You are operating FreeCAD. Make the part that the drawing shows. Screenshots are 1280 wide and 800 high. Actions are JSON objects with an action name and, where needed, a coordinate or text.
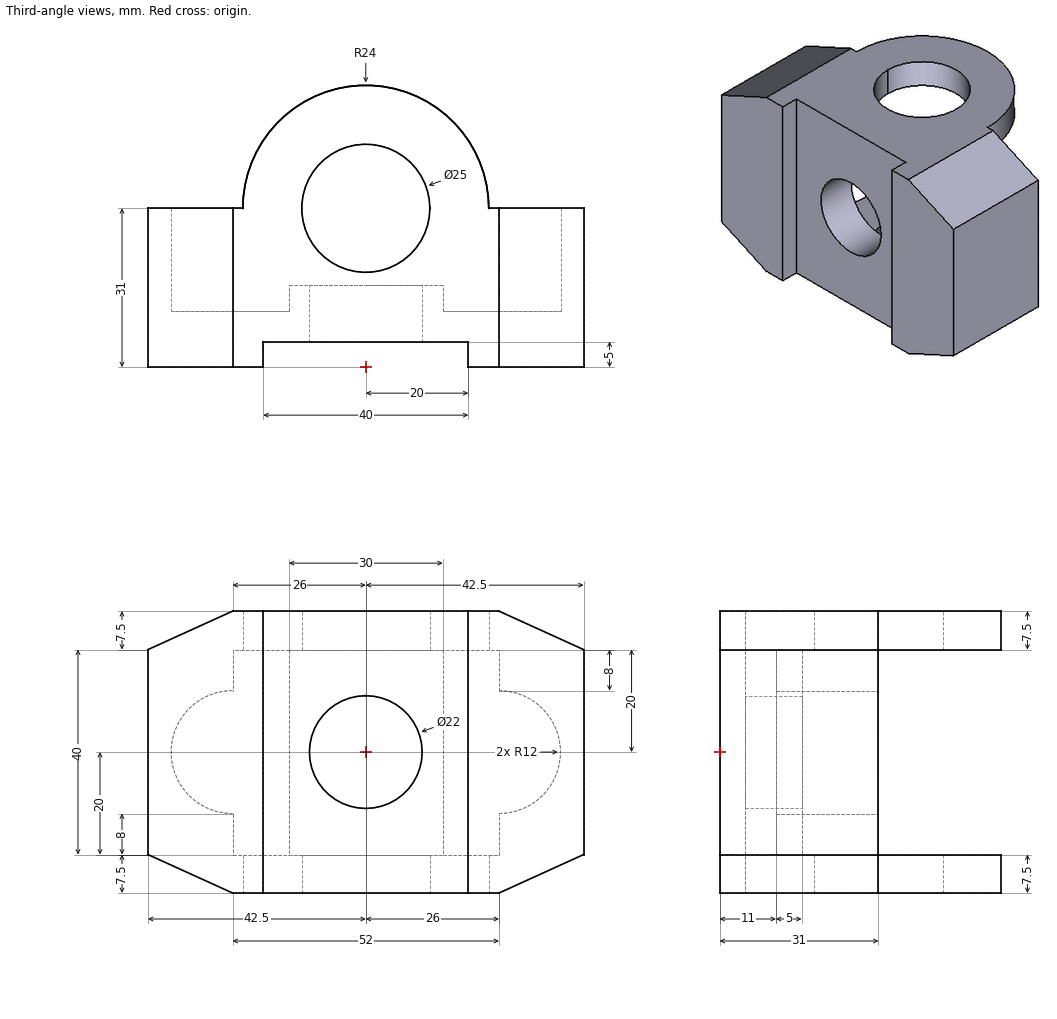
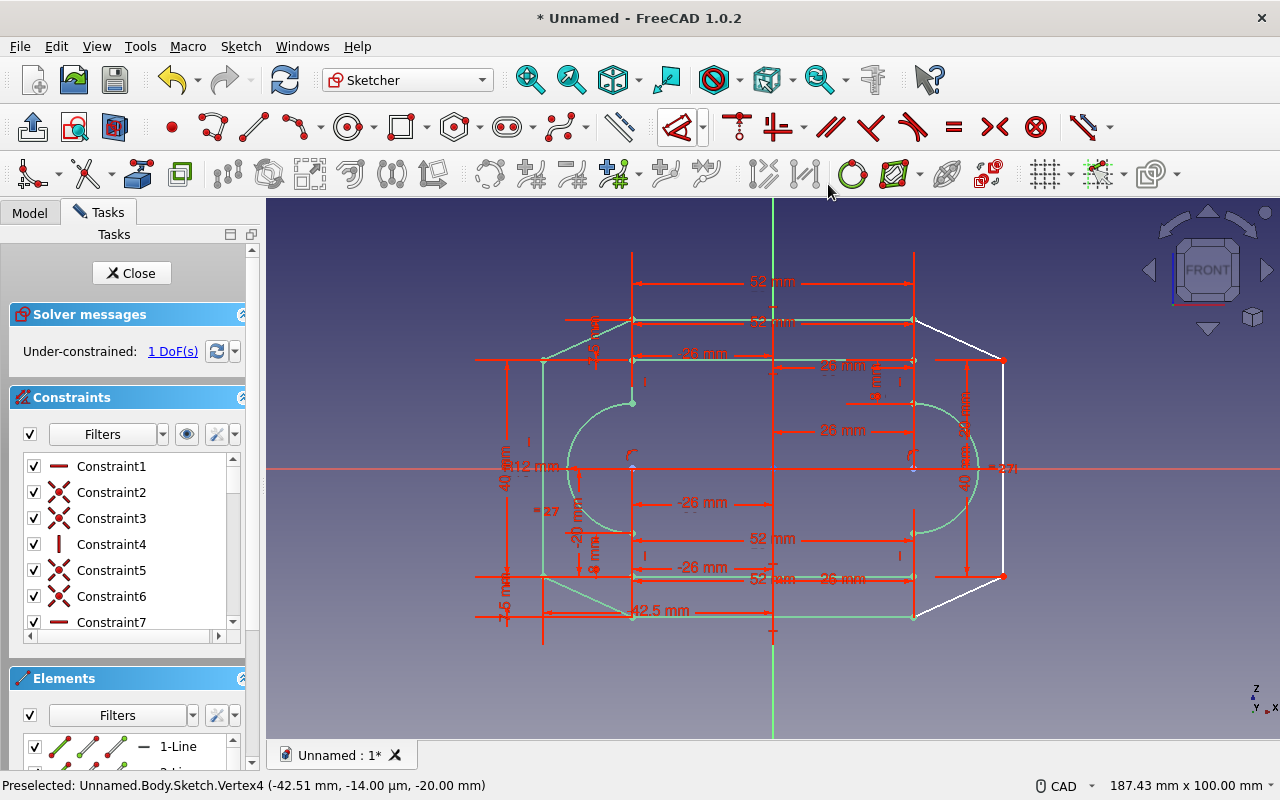
{"action": "left_click", "coordinate": [1003, 360]}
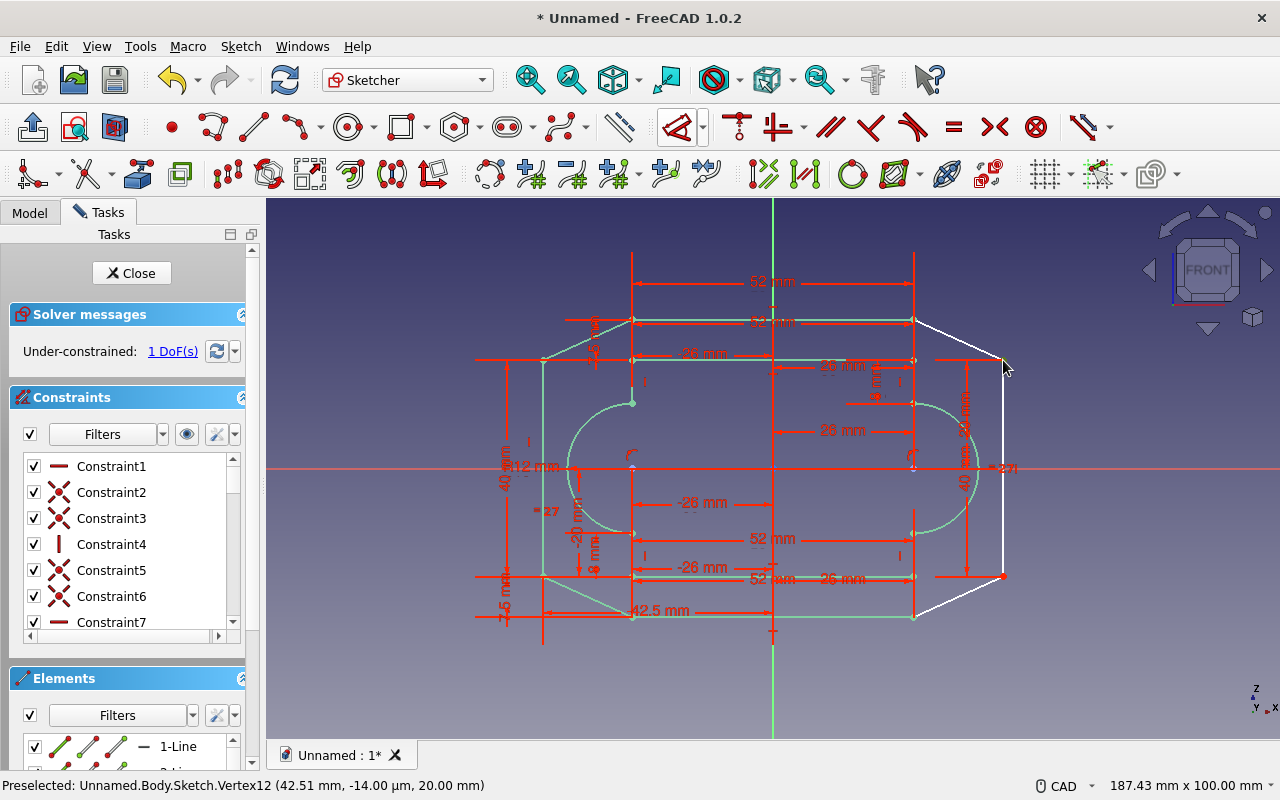
{"action": "left_click", "coordinate": [702, 128]}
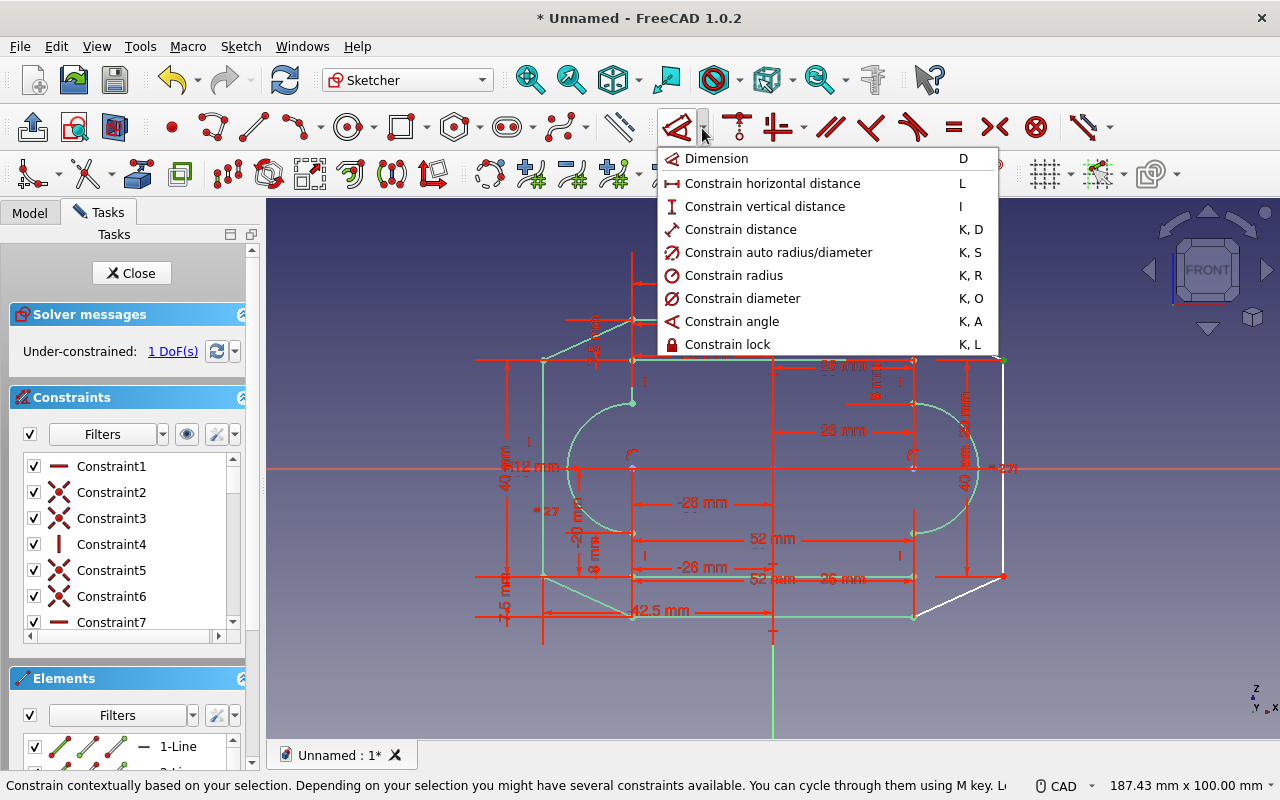
{"action": "left_click", "coordinate": [828, 184]}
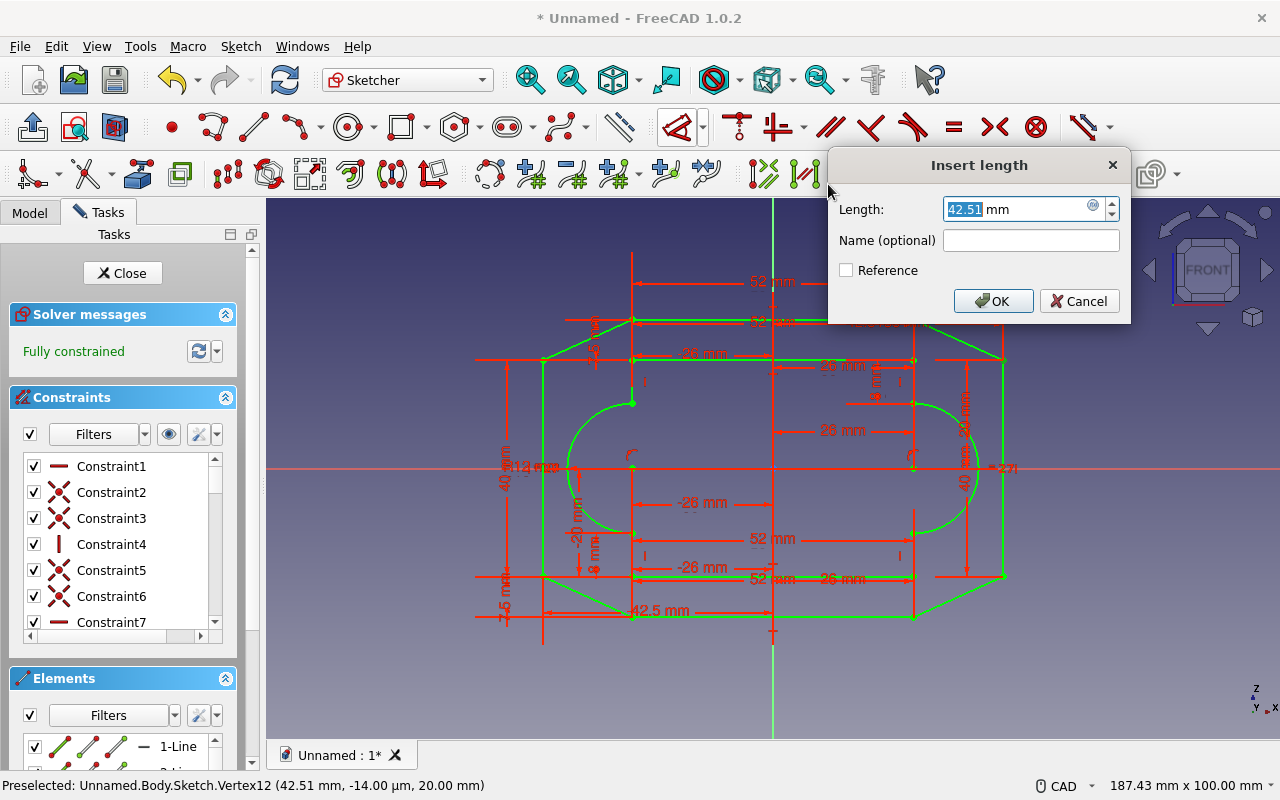
{"action": "type", "text": "42.5"}
{"action": "key", "text": "Return"}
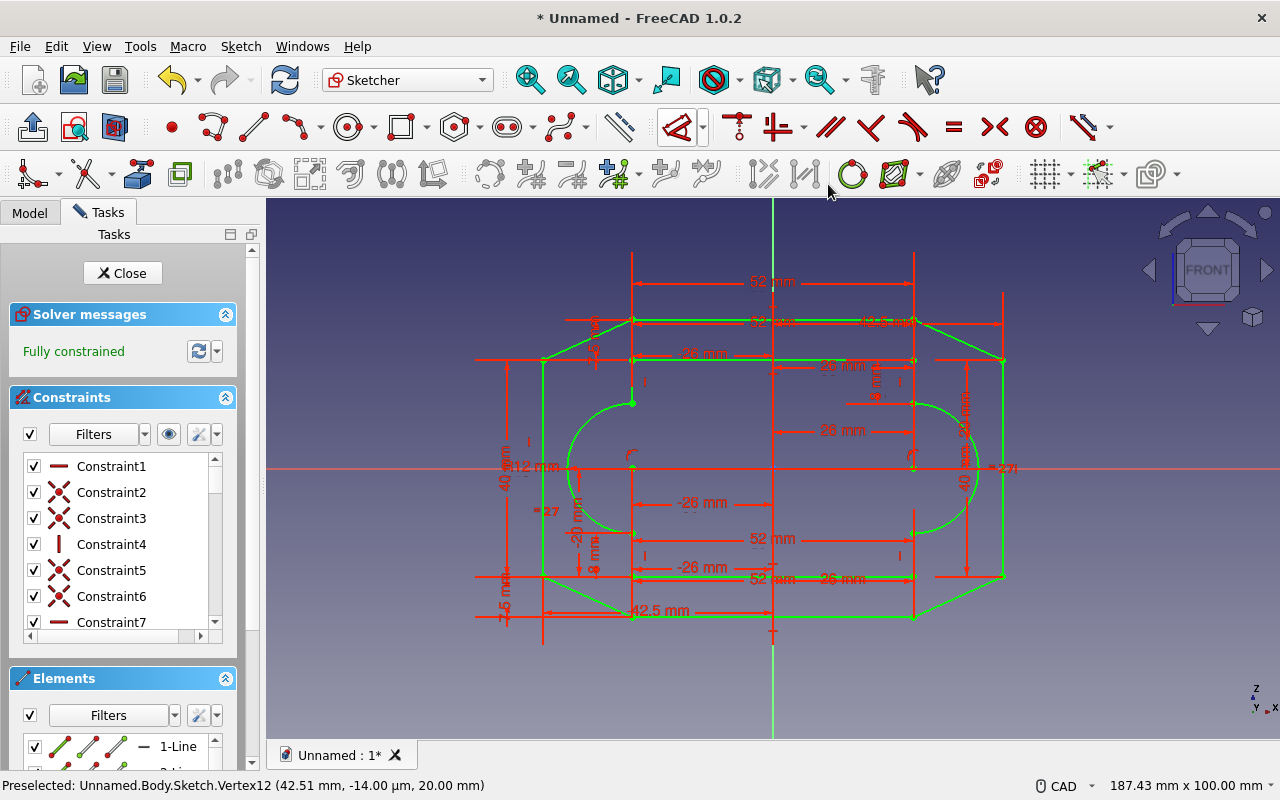
{"action": "left_click", "coordinate": [123, 273]}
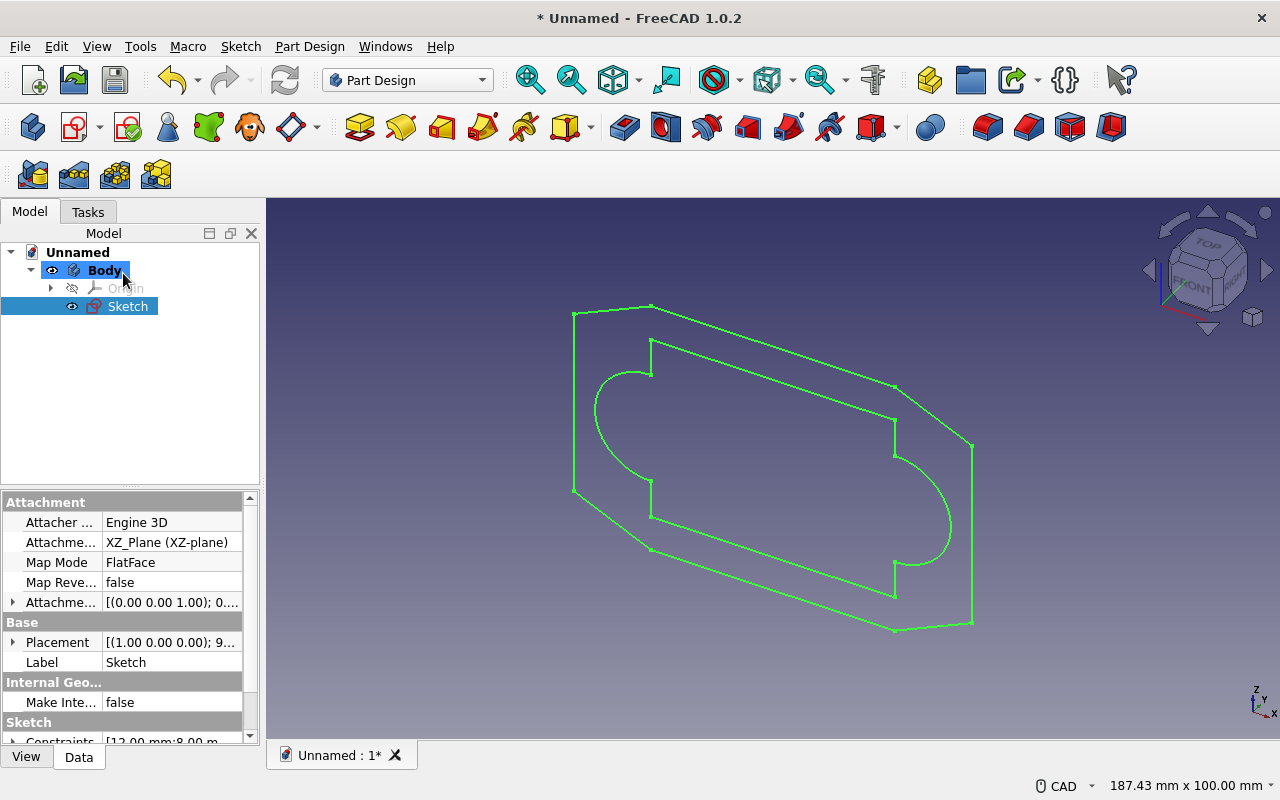
{"action": "left_click", "coordinate": [360, 128]}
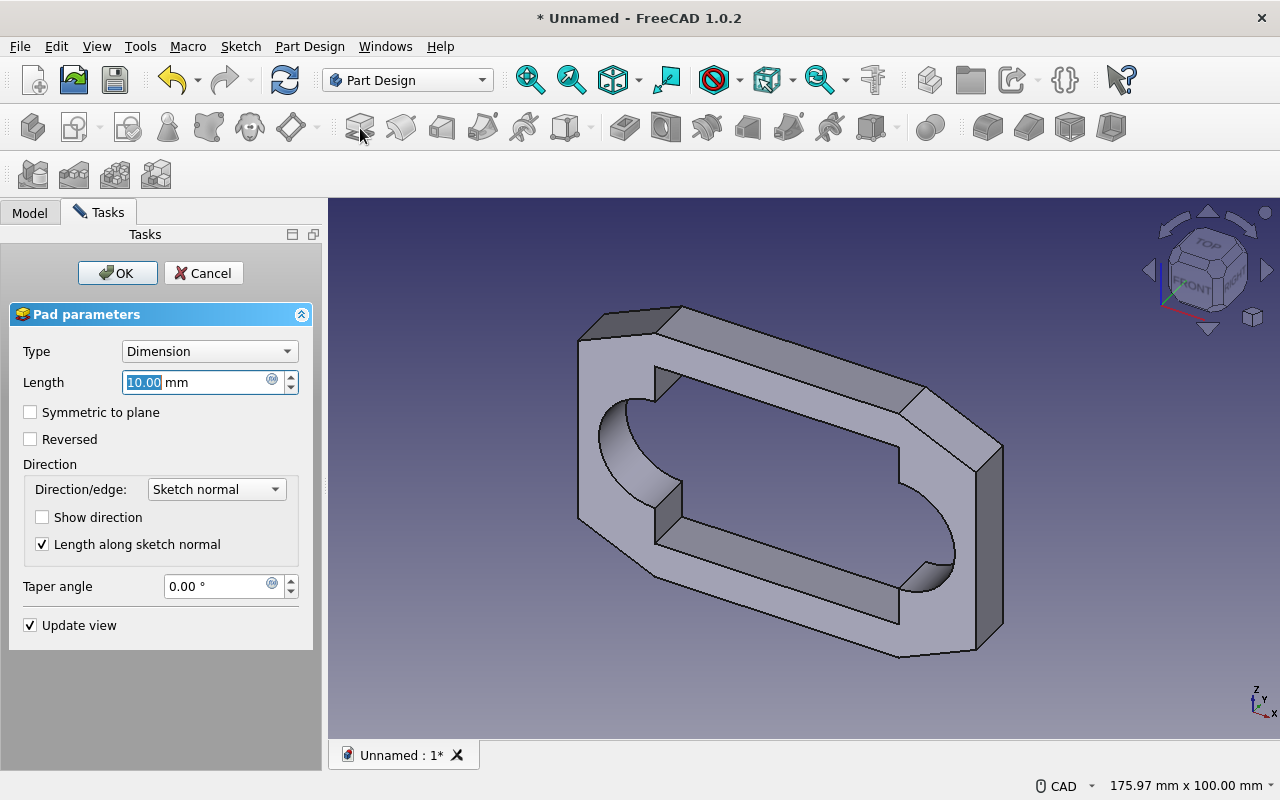
{"action": "type", "text": "31"}
{"action": "key", "text": "Tab"}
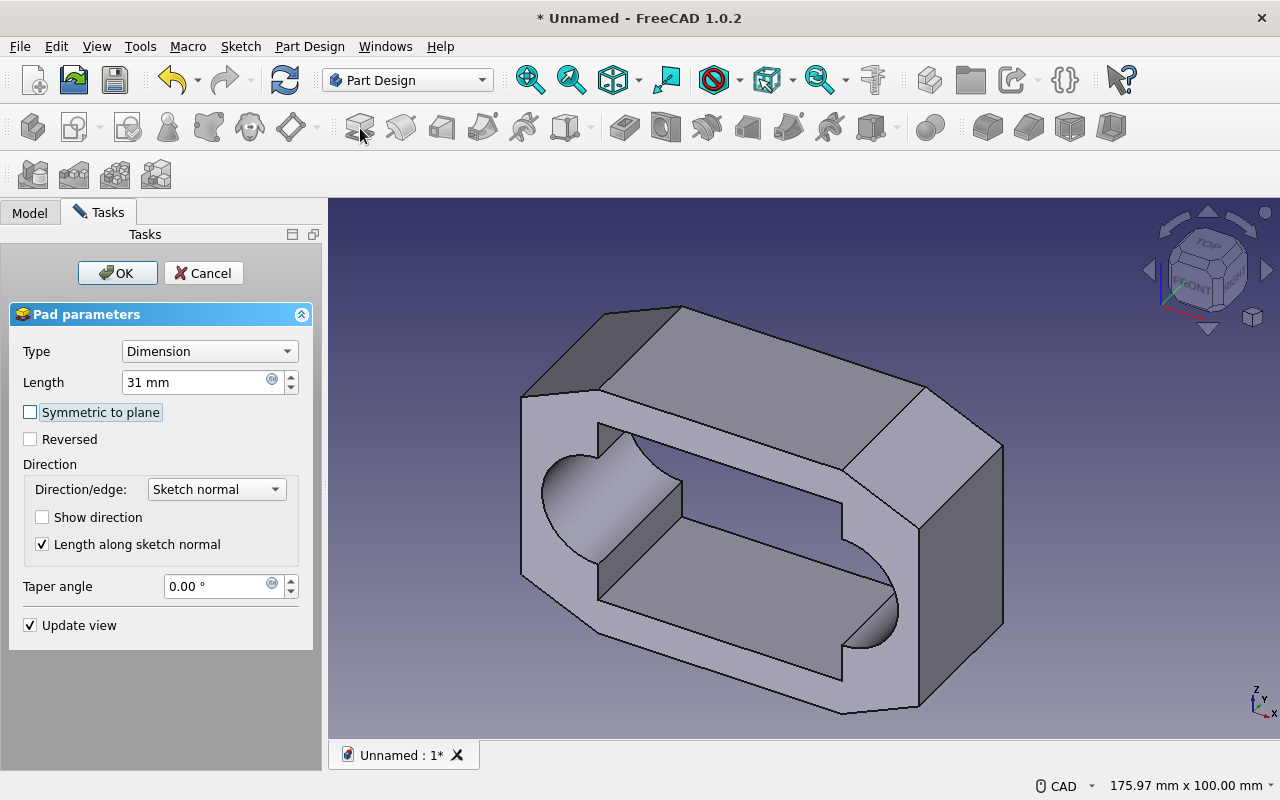
{"action": "left_click", "coordinate": [31, 439]}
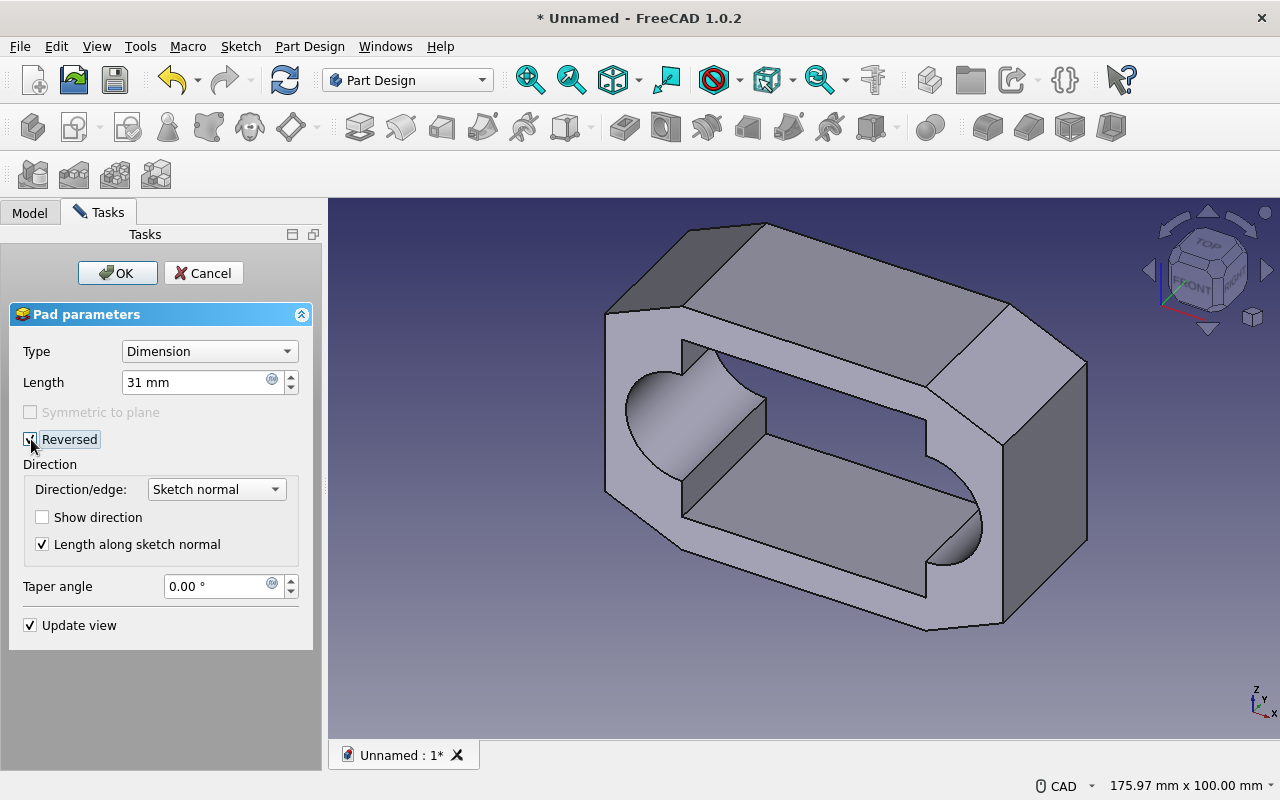
{"action": "left_click", "coordinate": [118, 273]}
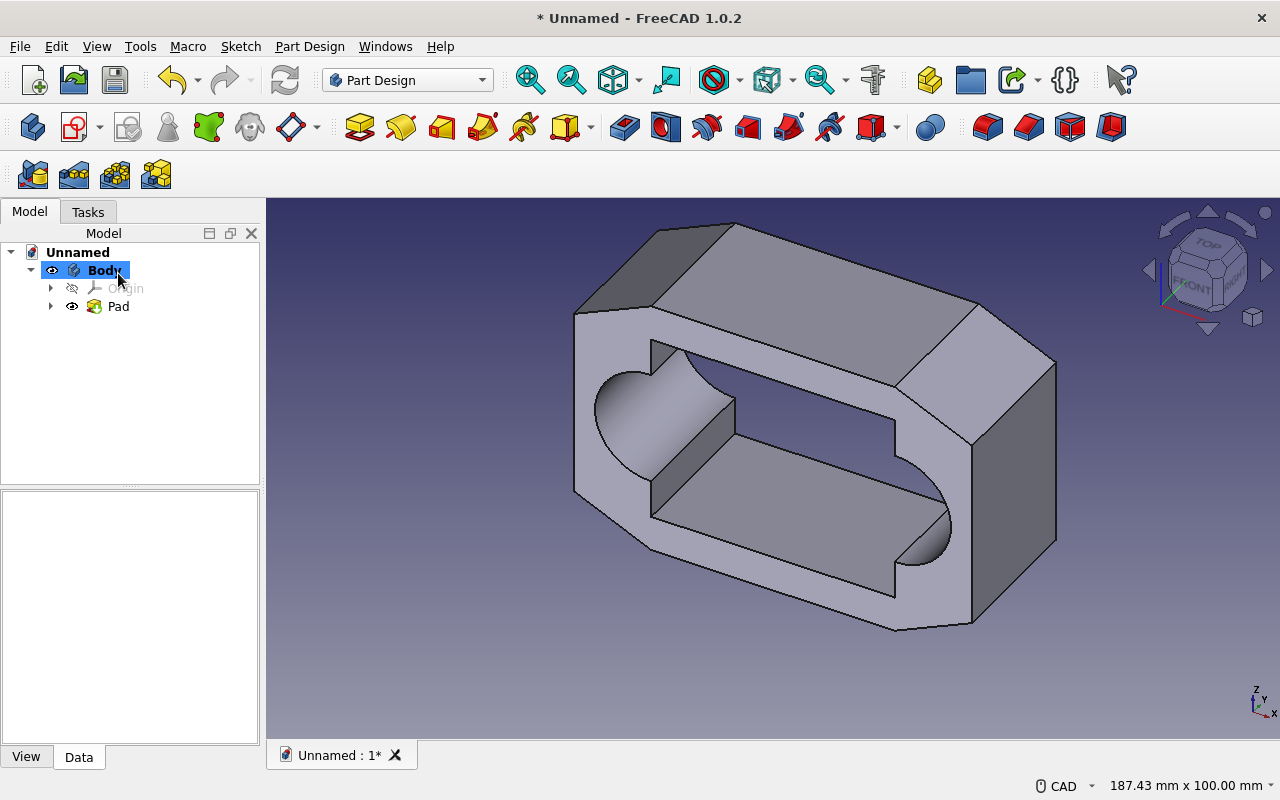
{"action": "key", "text": "v f"}